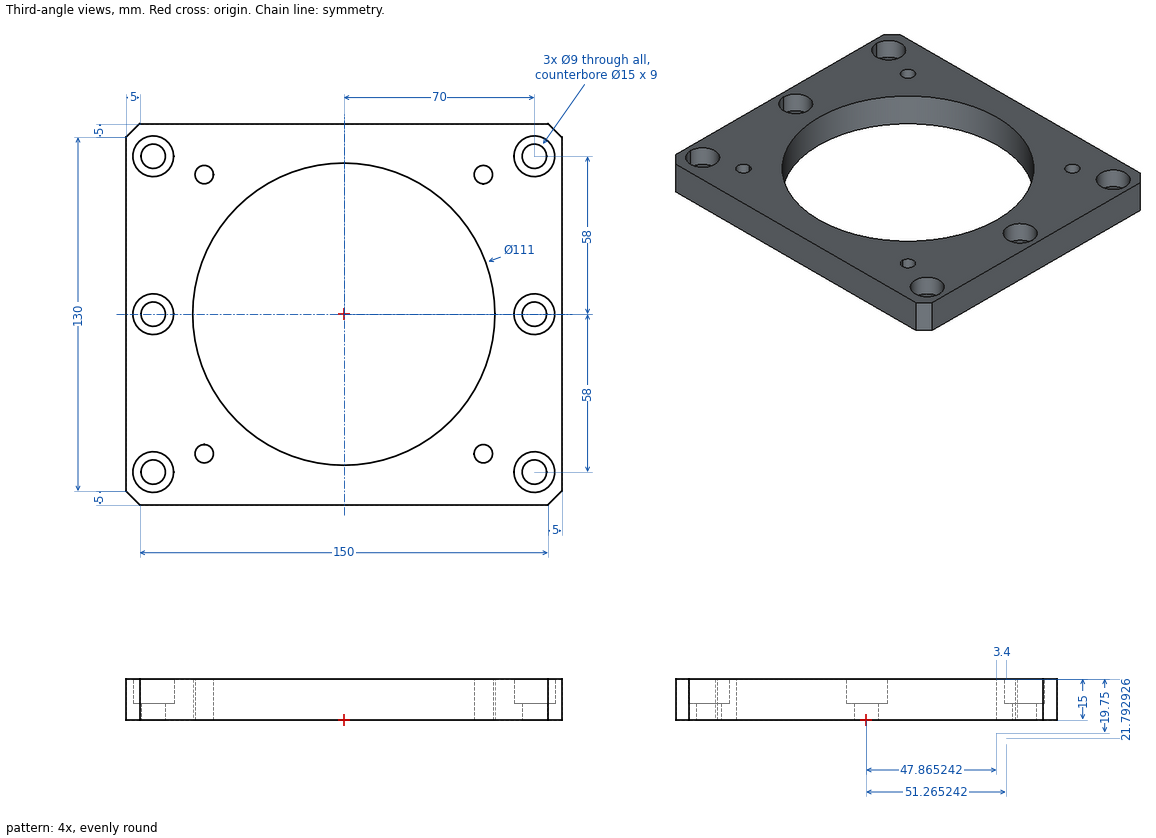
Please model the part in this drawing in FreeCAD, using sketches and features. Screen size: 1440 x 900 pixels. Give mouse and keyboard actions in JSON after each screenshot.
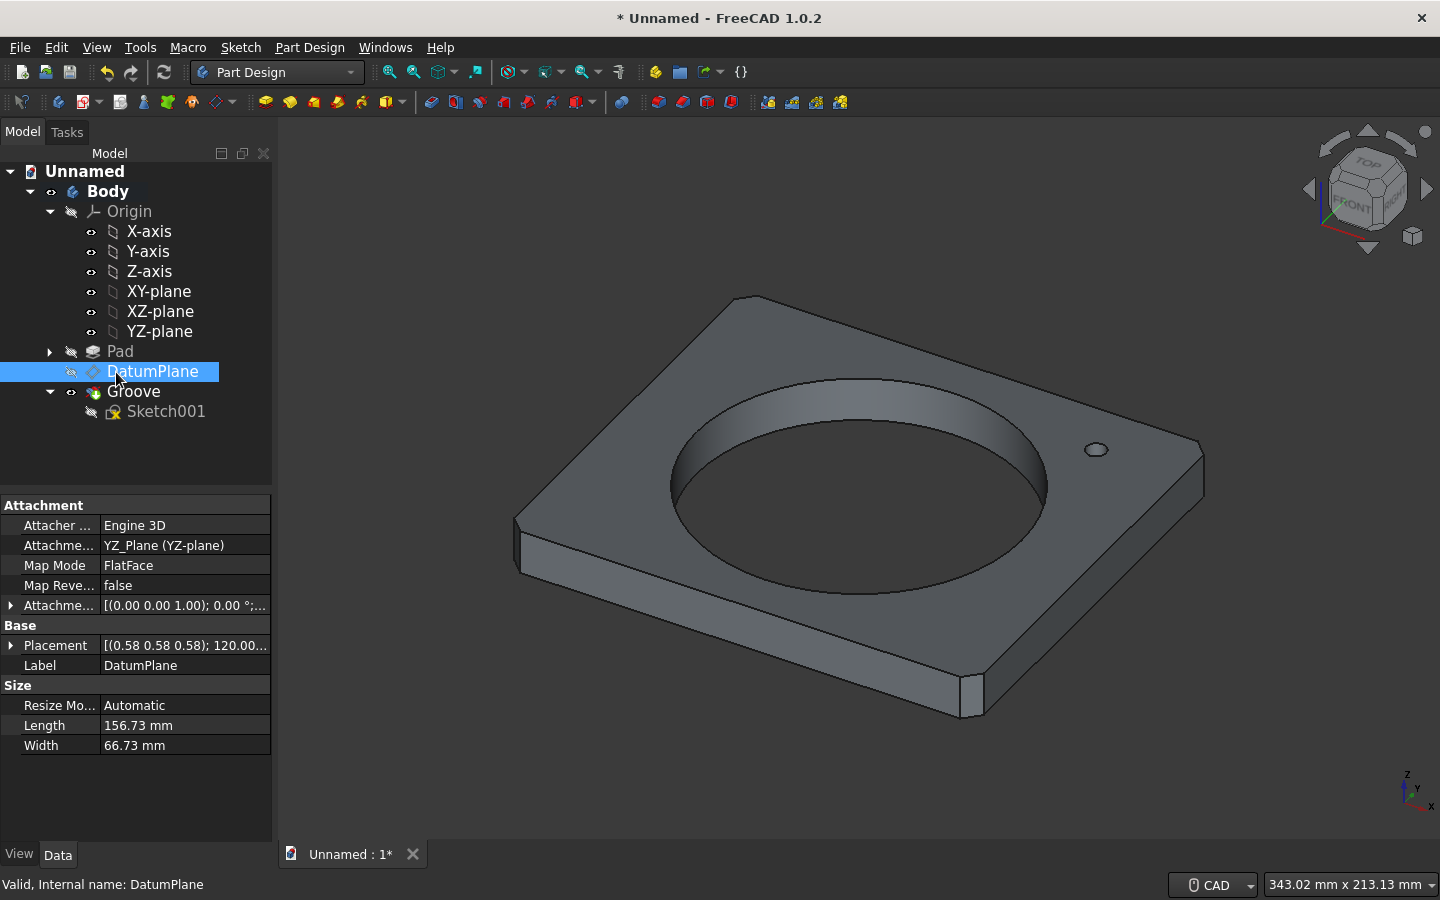
{"action": "left_click", "coordinate": [116, 392]}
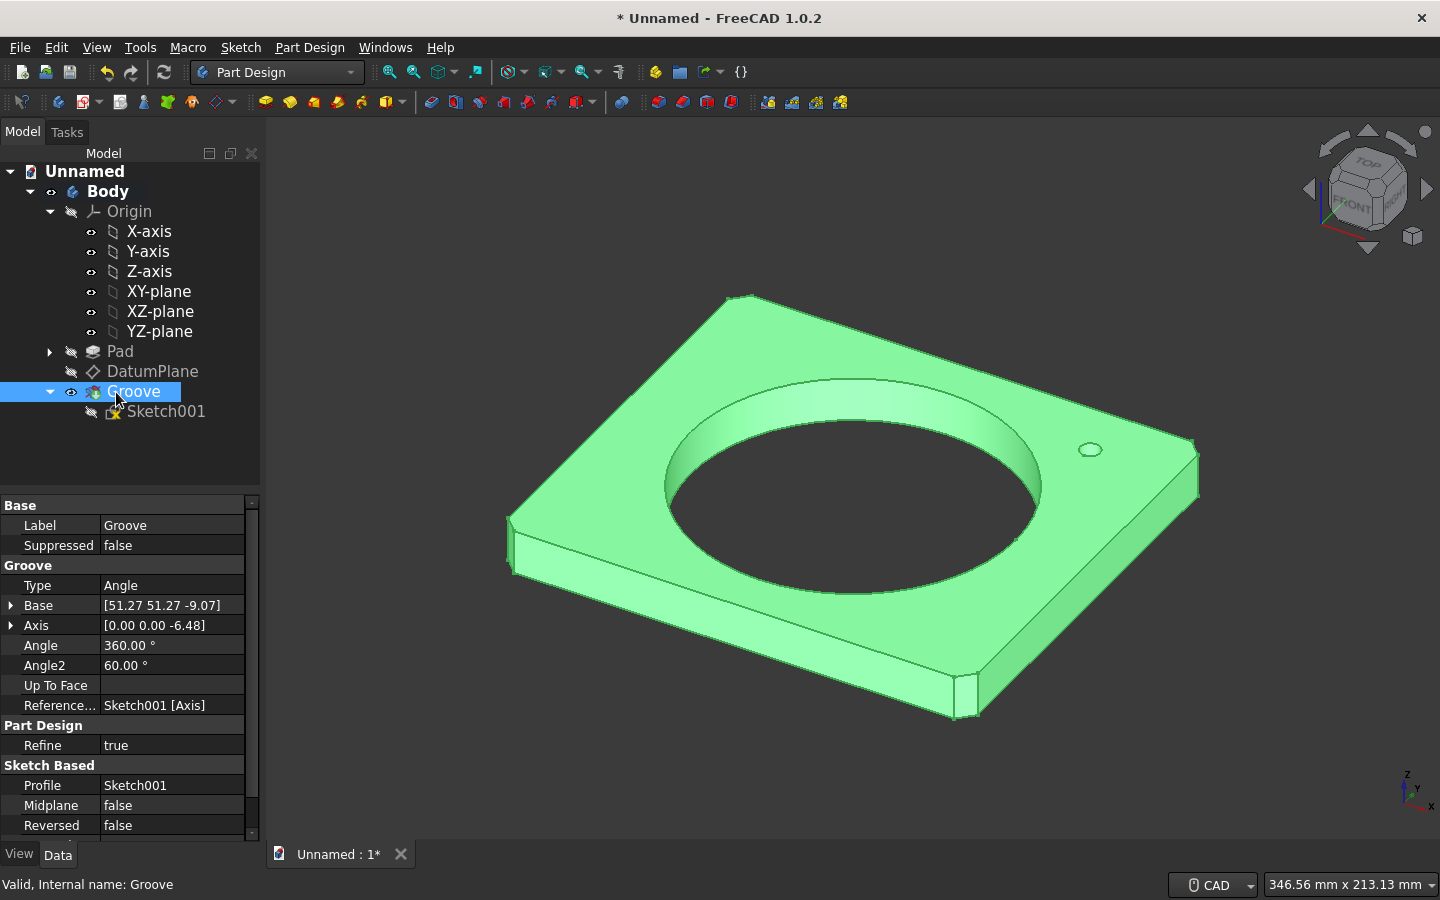
{"action": "left_click", "coordinate": [816, 102]}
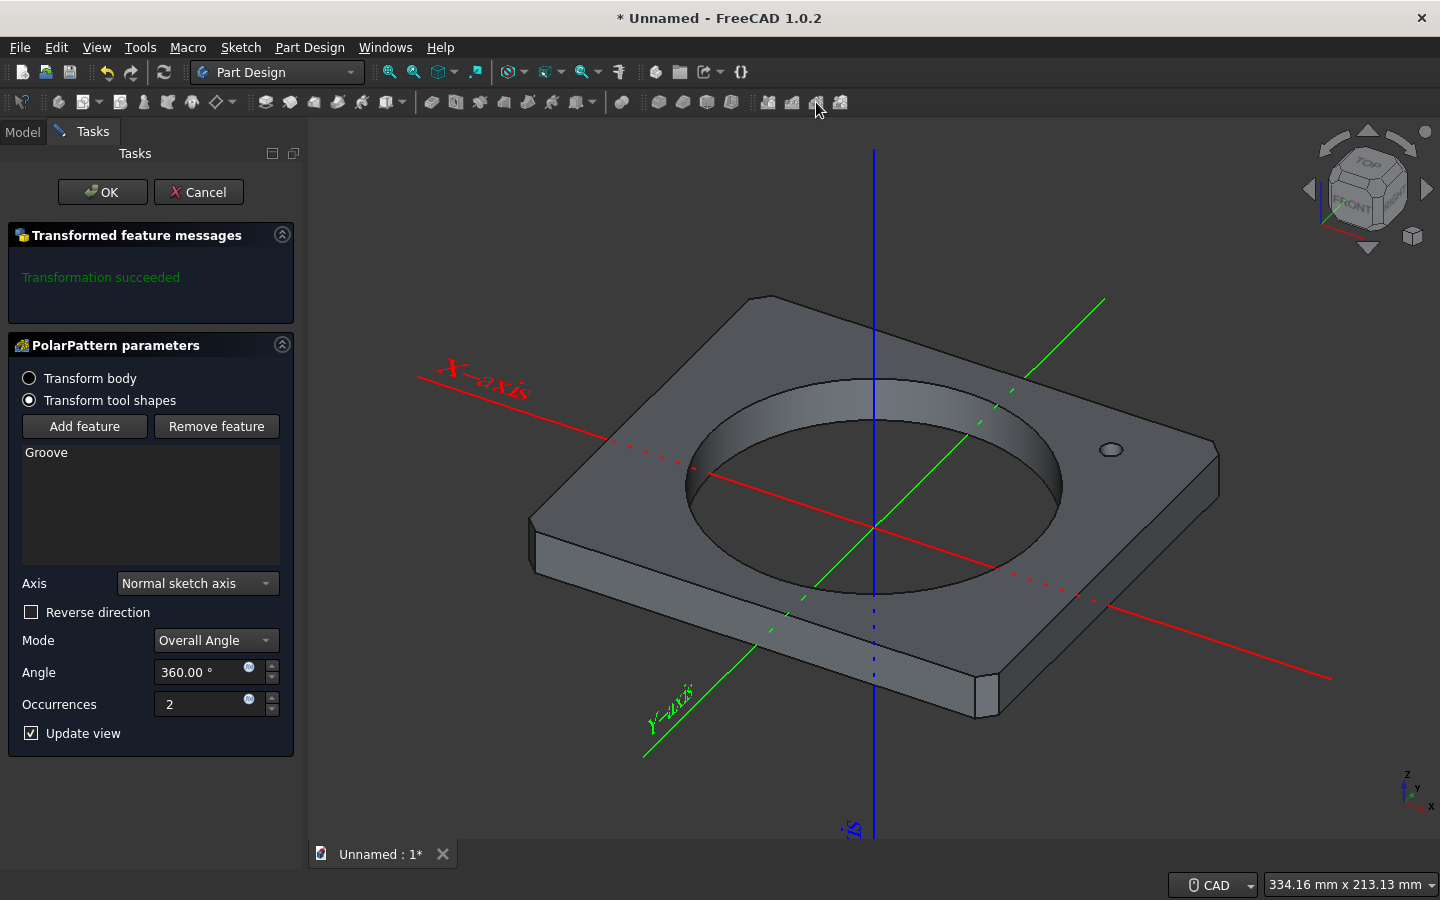
{"action": "left_click", "coordinate": [198, 584]}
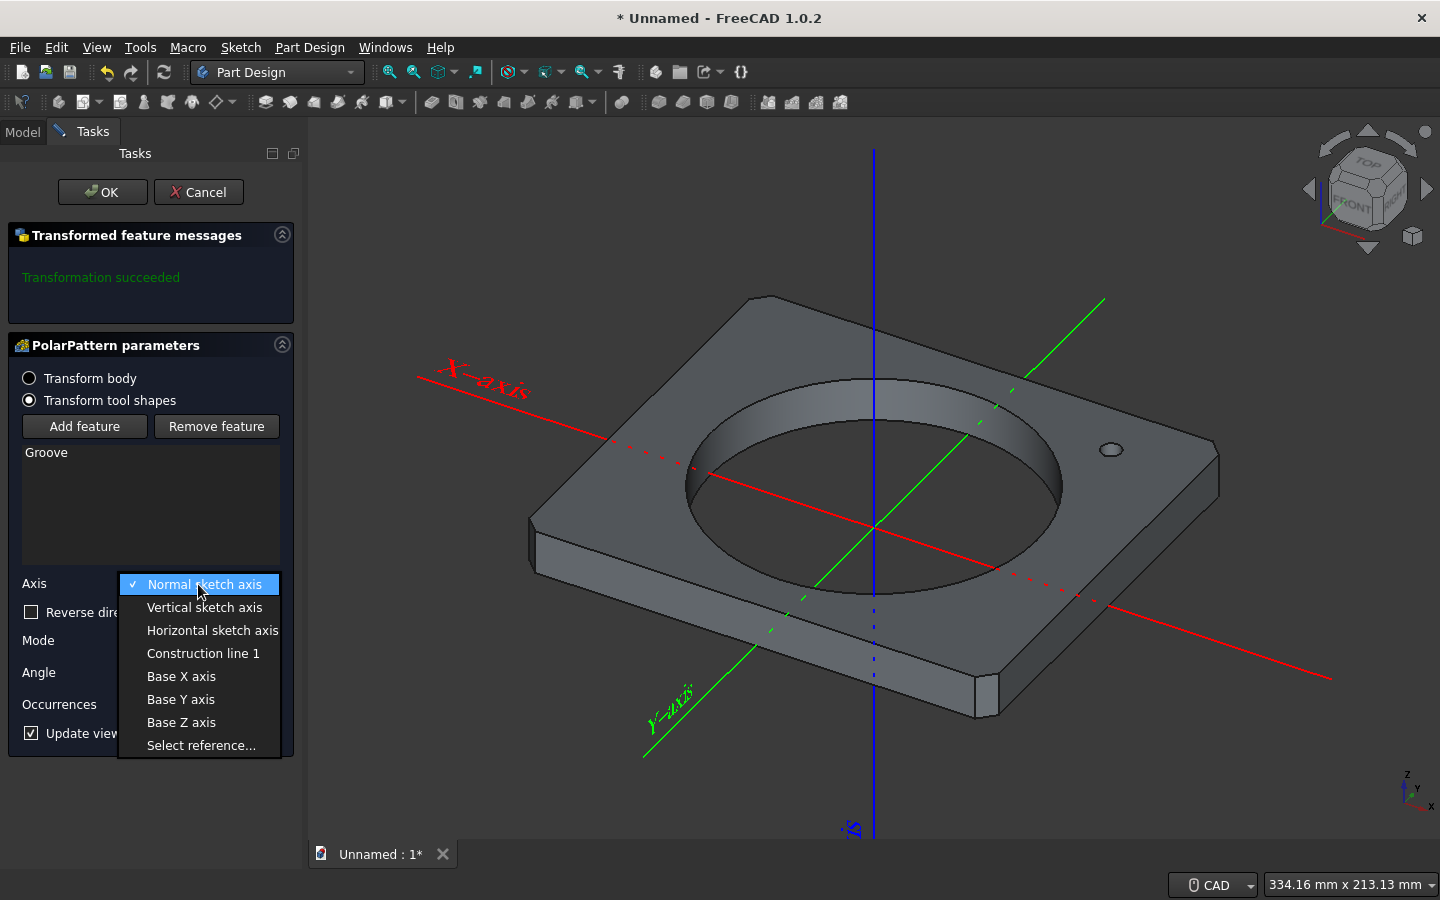
{"action": "left_click", "coordinate": [198, 722]}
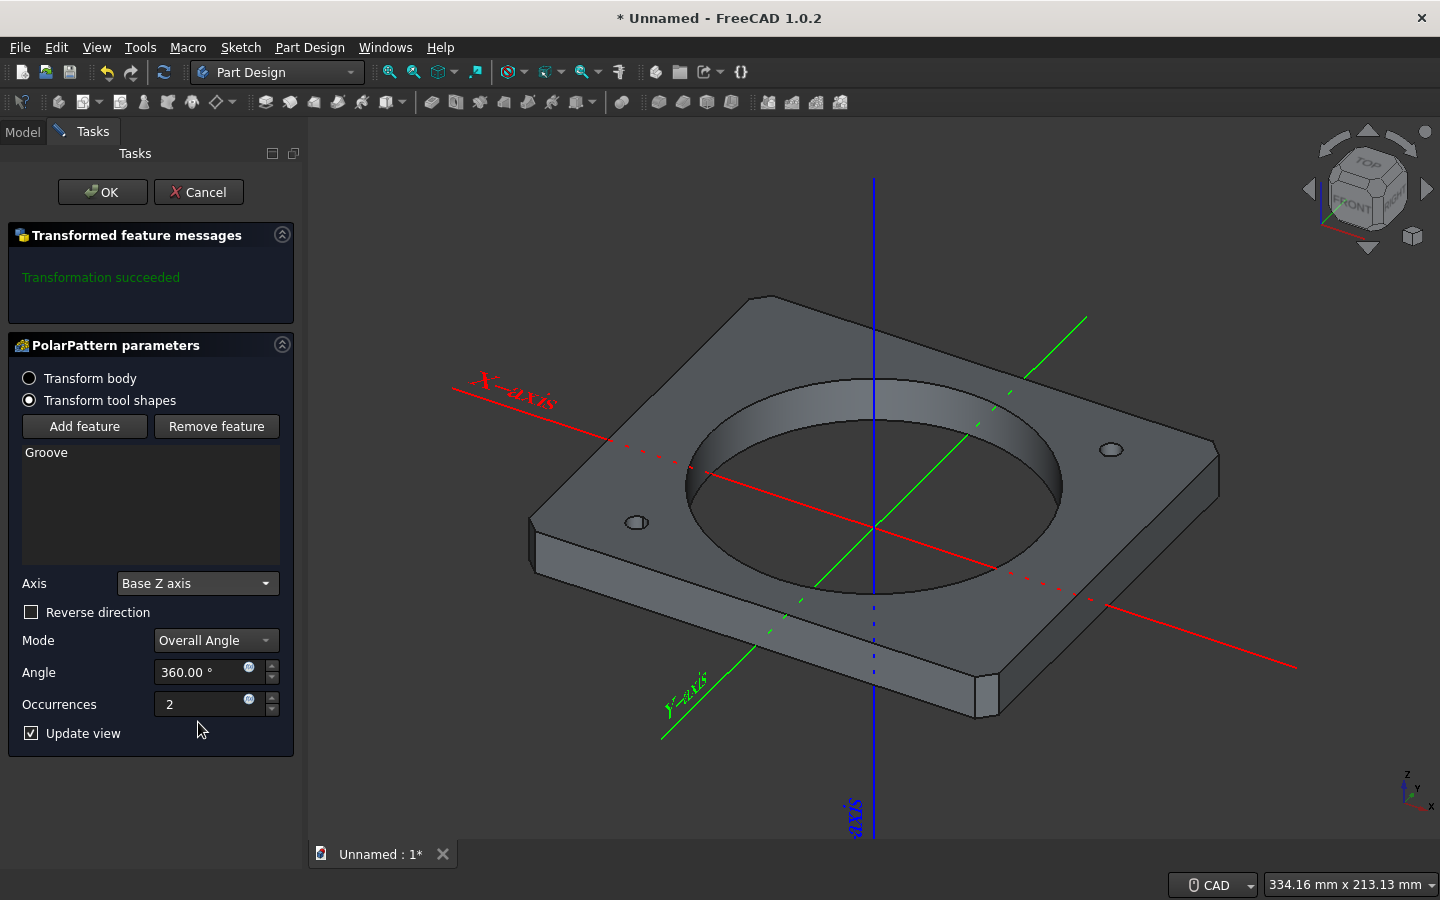
{"action": "triple_click", "coordinate": [209, 704]}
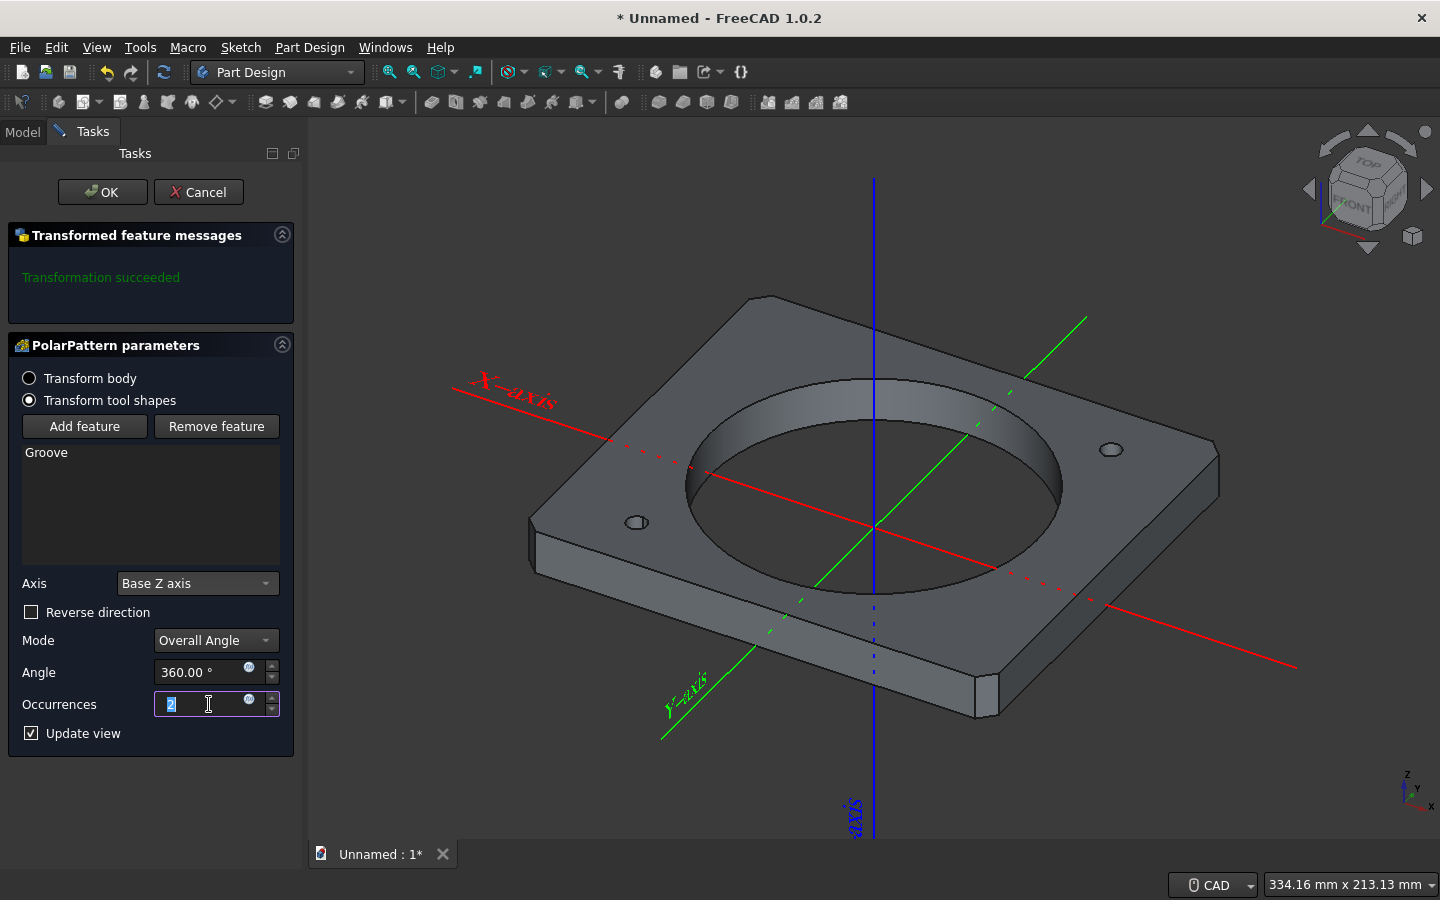
{"action": "type", "text": "4"}
{"action": "key", "text": "Tab"}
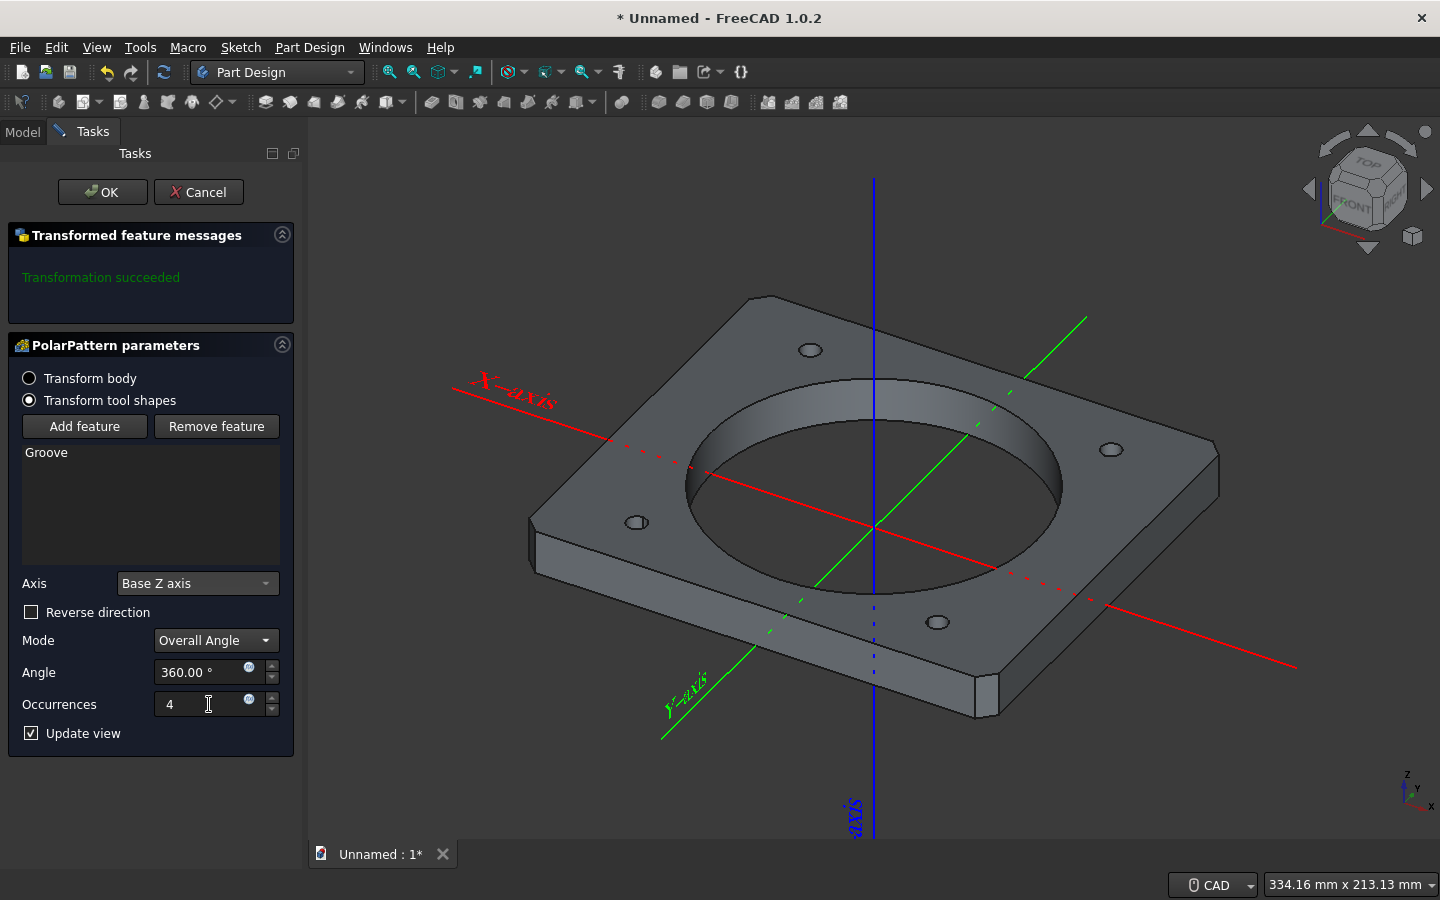
{"action": "left_click", "coordinate": [103, 192]}